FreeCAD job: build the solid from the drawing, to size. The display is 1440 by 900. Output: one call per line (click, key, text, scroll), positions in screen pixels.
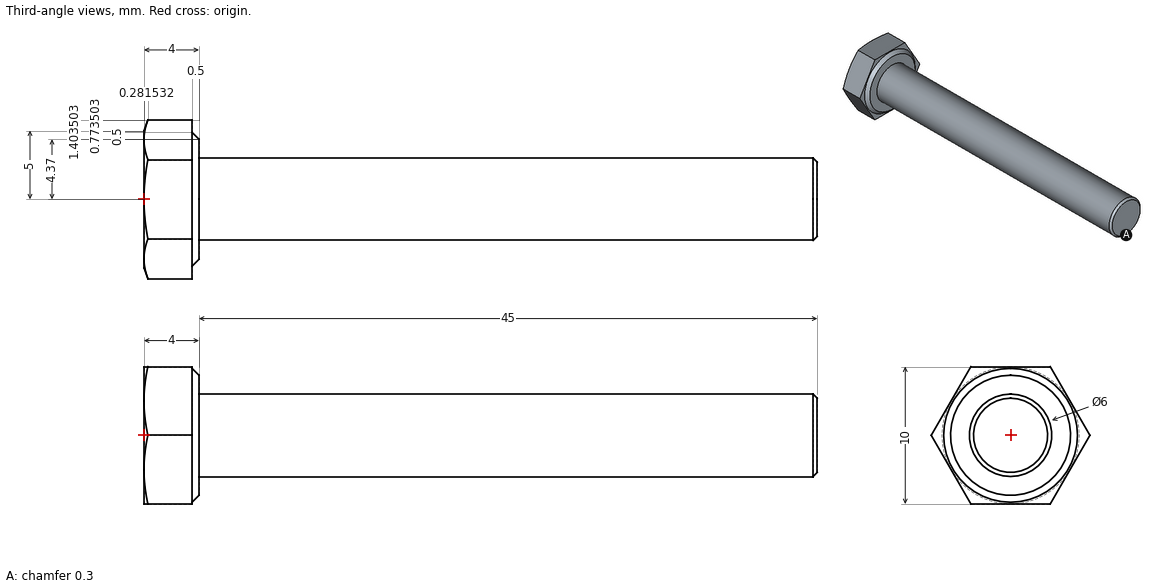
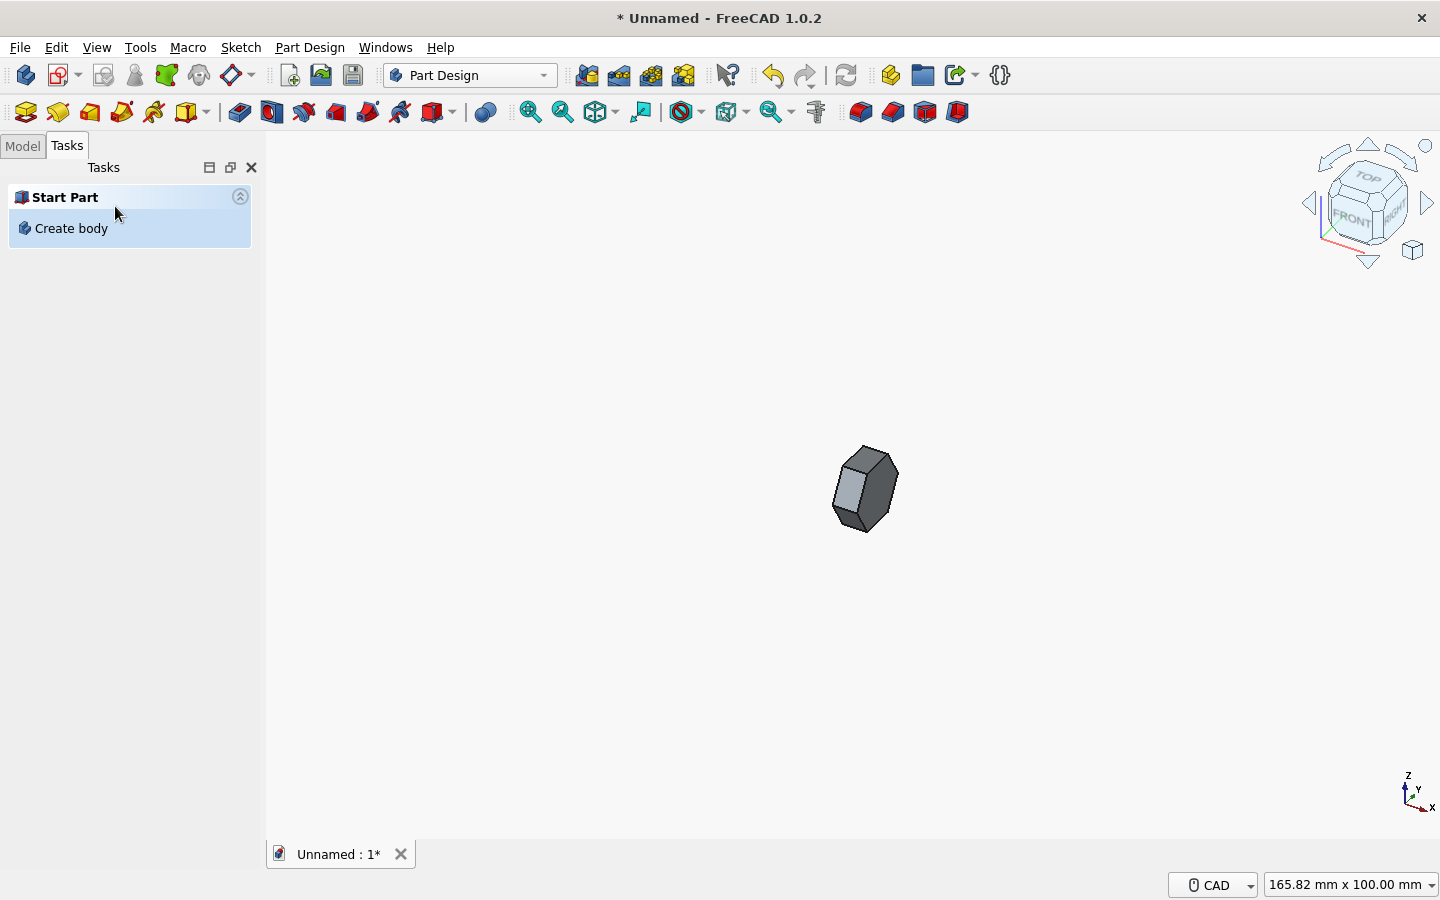
click(532, 112)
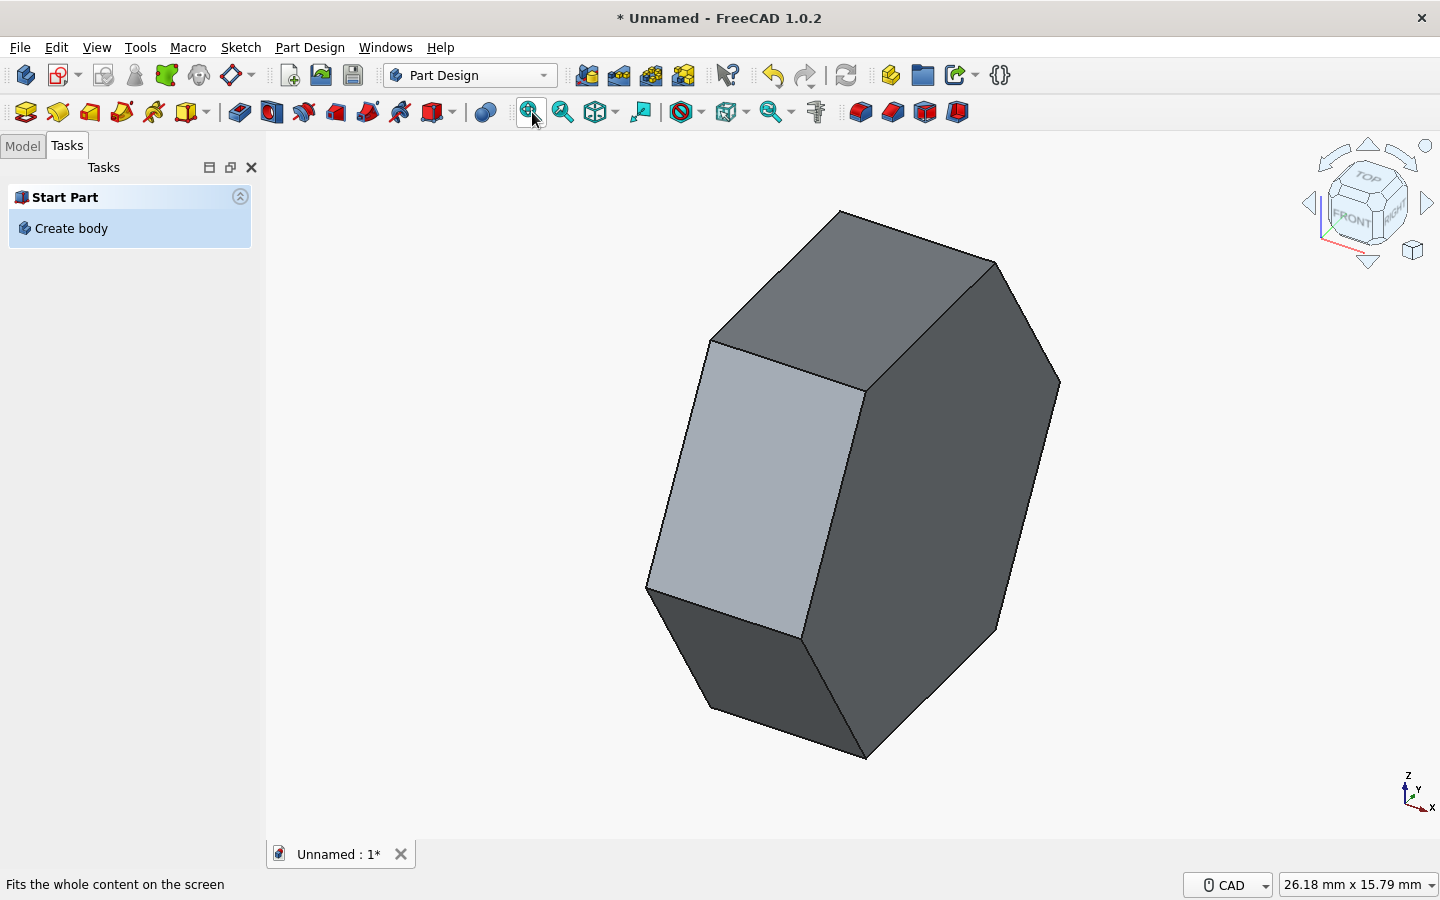
click(58, 76)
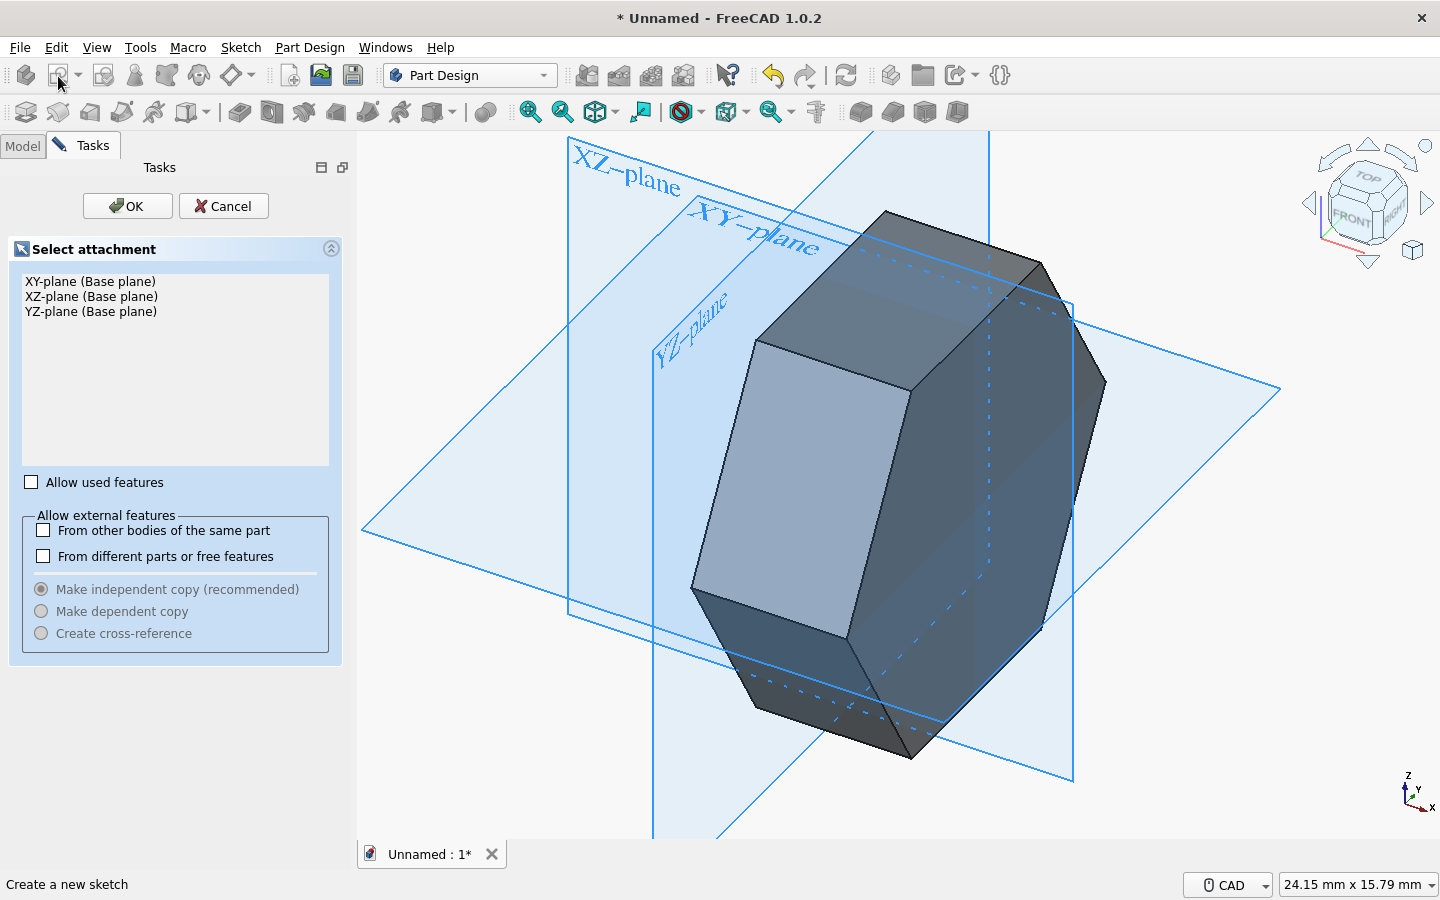
click(82, 282)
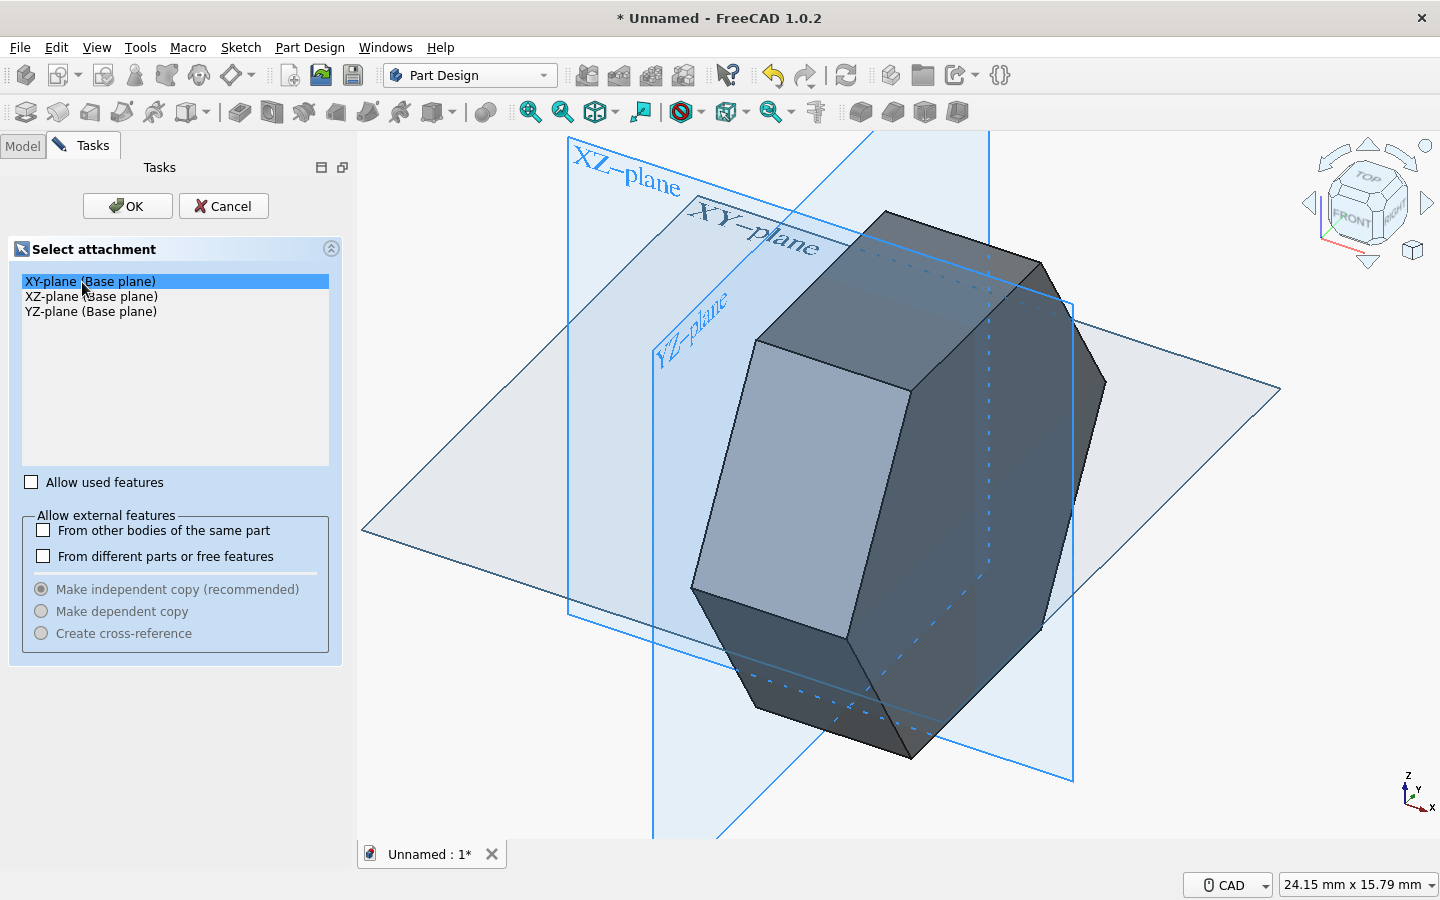
click(128, 206)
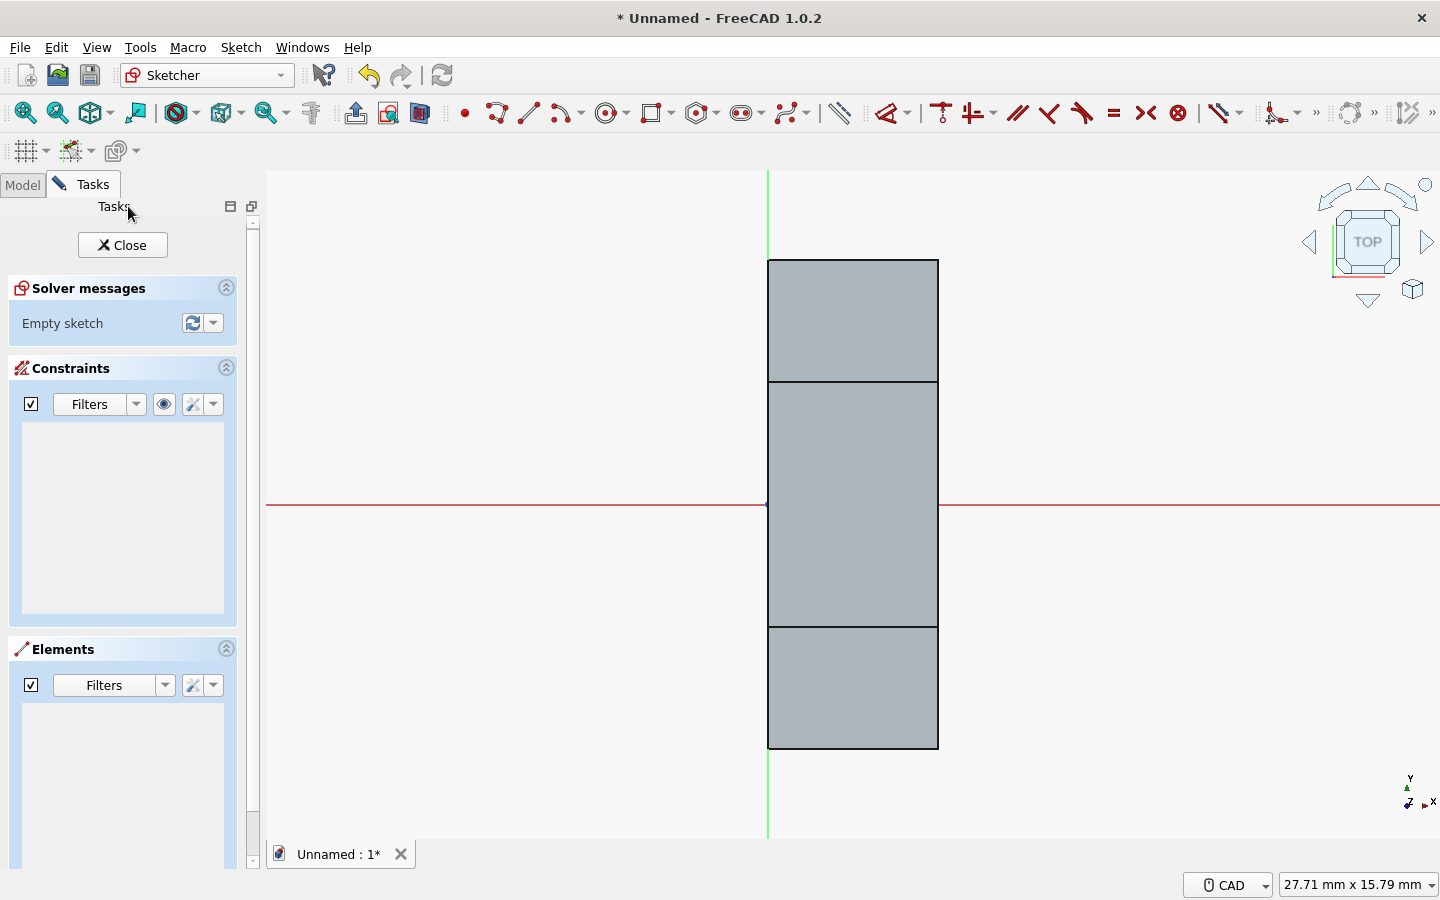
click(420, 114)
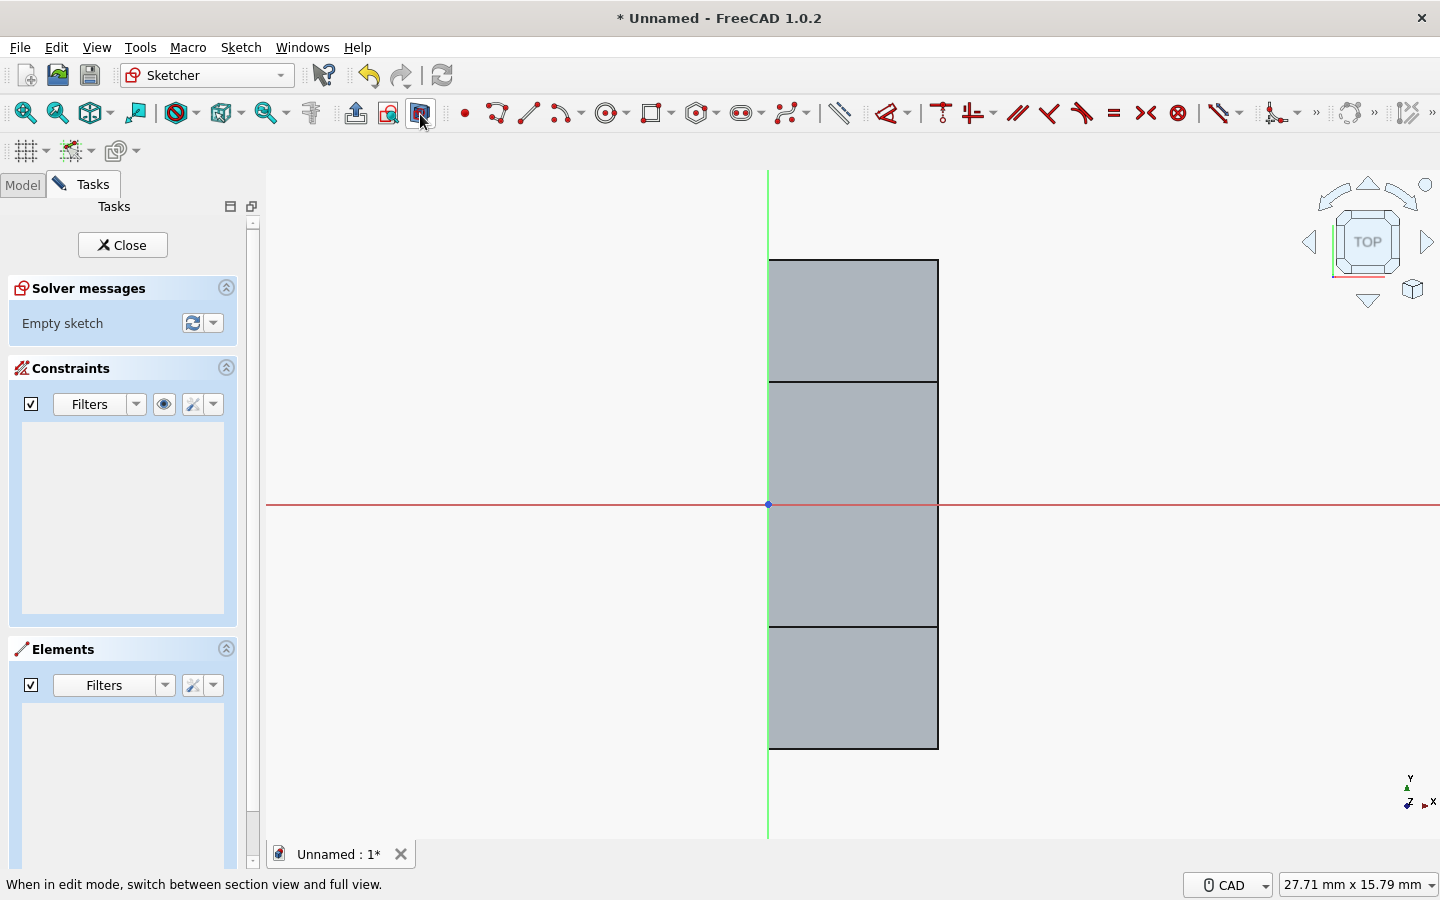
scroll(949, 256, up, 10)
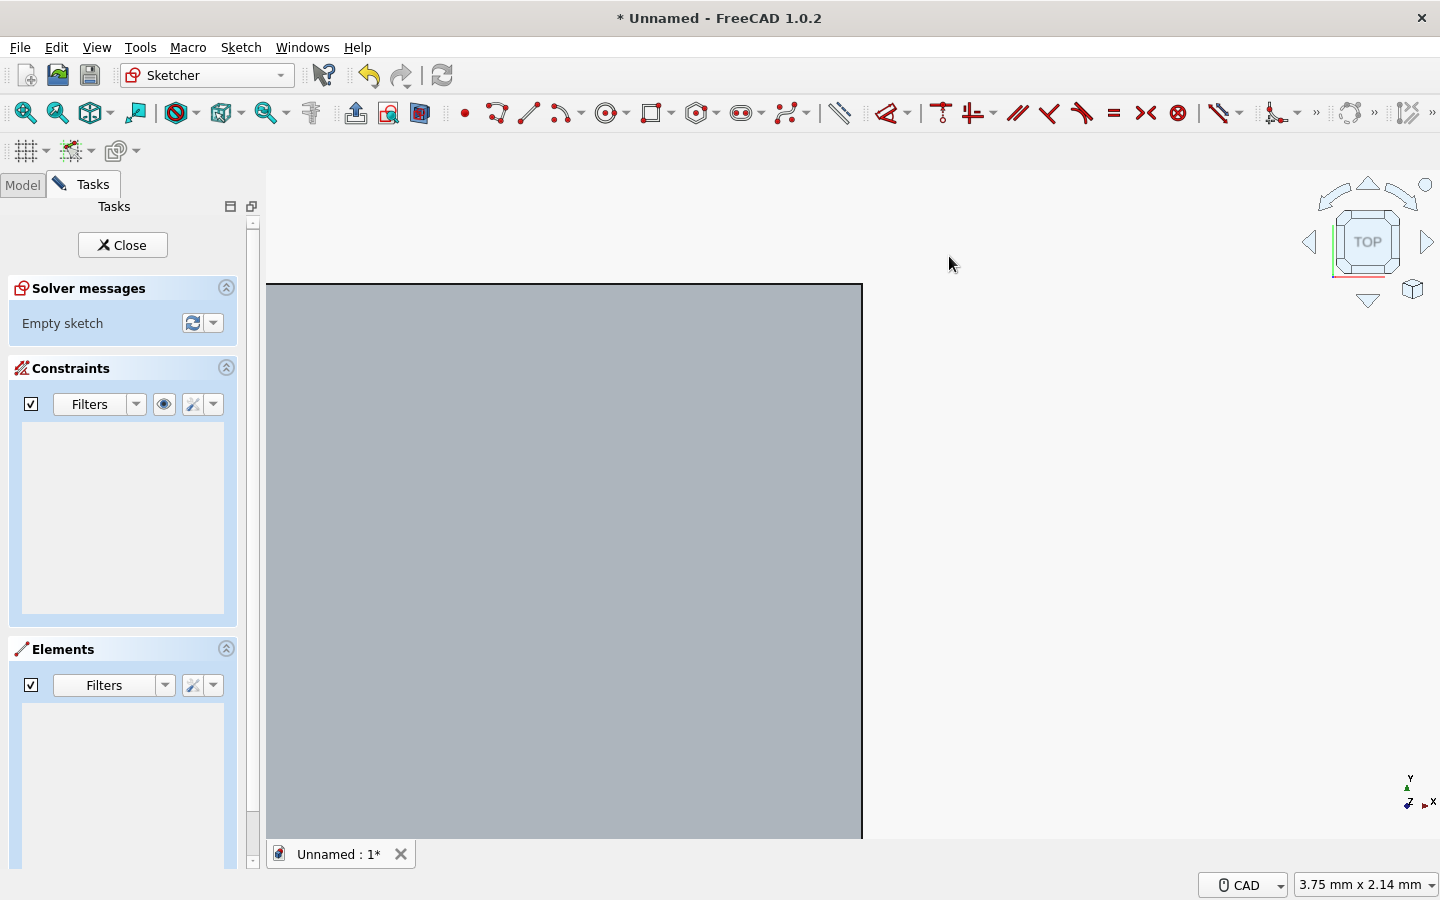
click(498, 114)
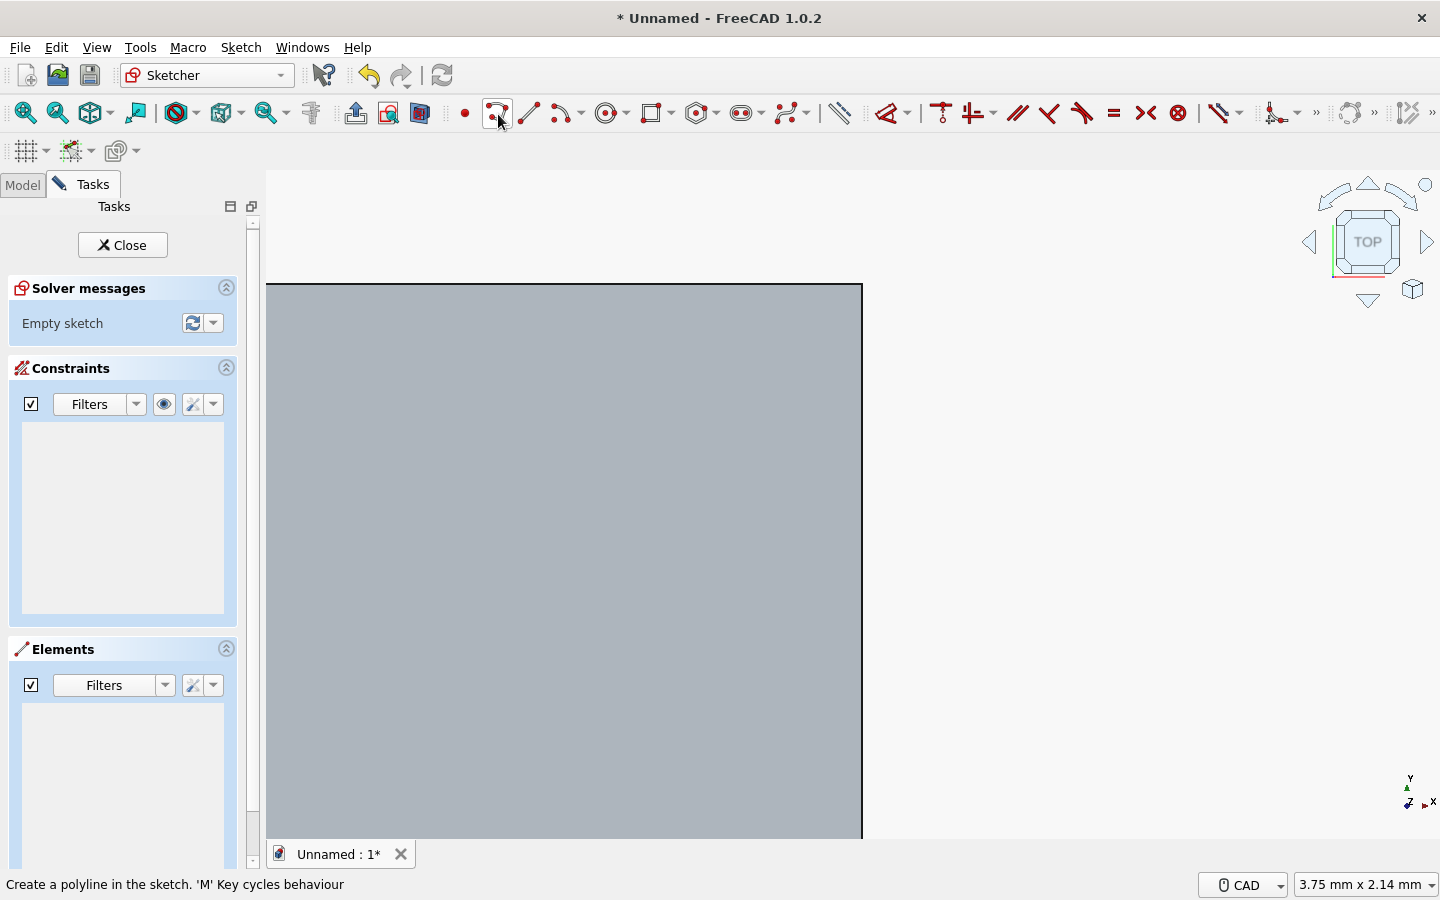
click(862, 723)
click(862, 284)
click(706, 284)
click(706, 567)
click(862, 724)
key(Escape)
key(Escape)